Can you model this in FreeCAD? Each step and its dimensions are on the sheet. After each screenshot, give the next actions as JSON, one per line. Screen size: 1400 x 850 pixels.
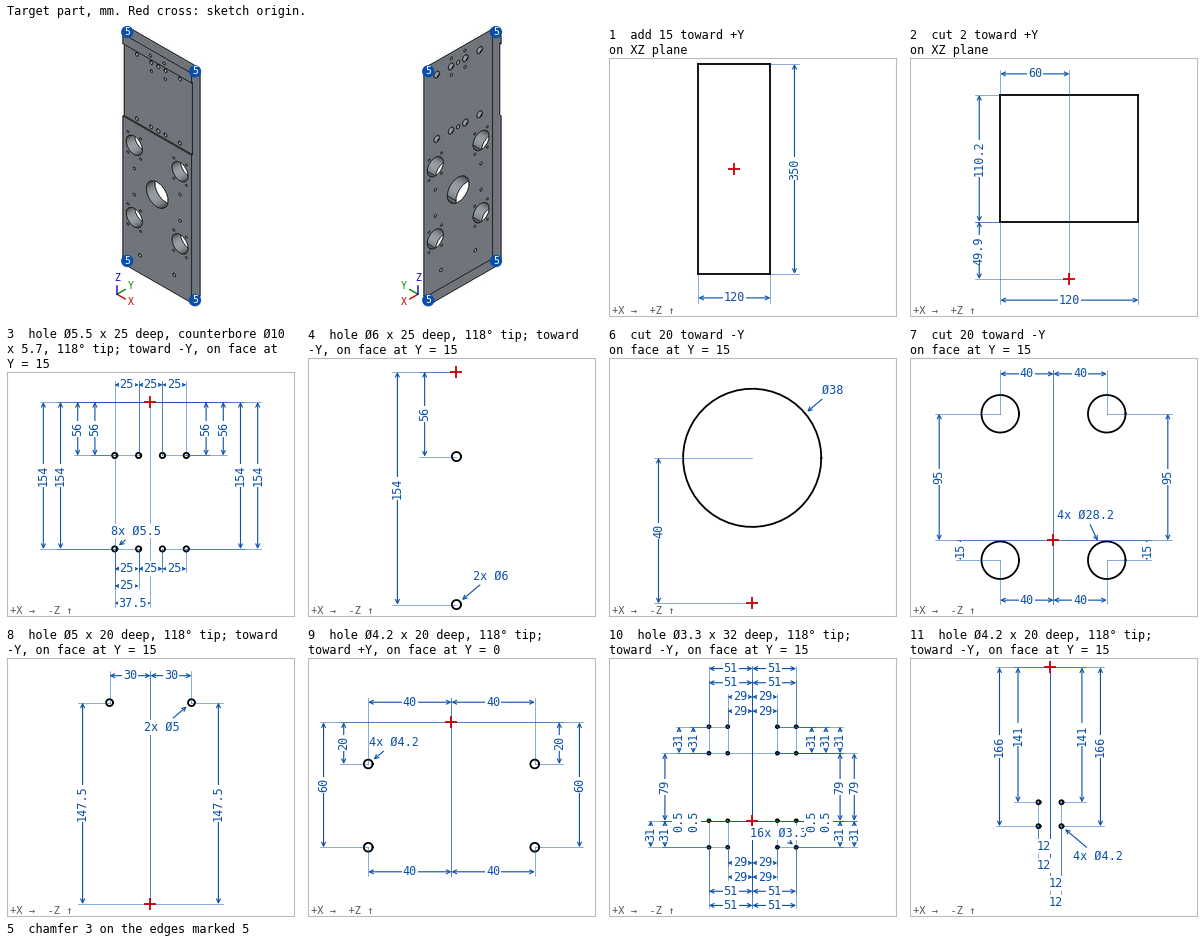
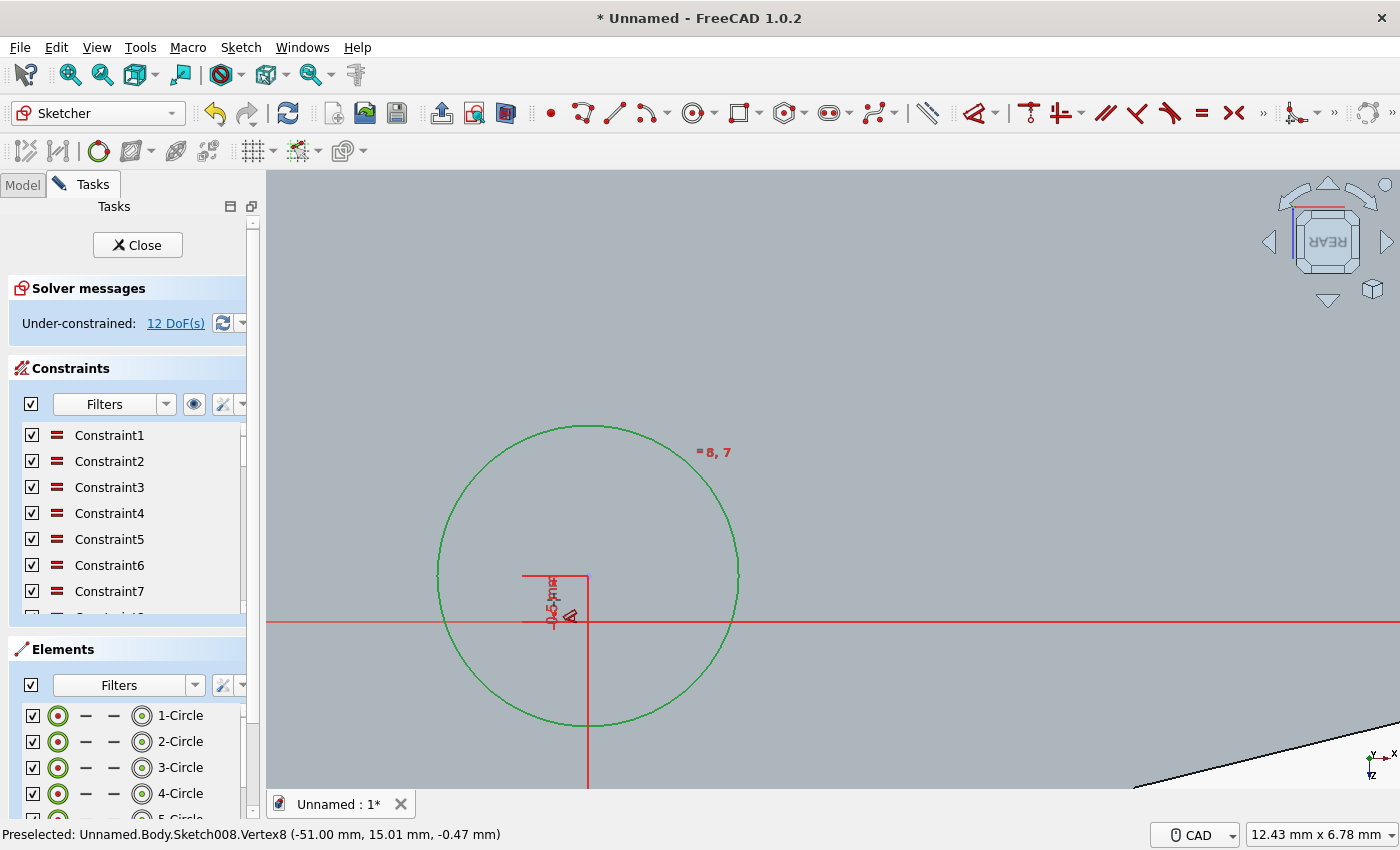
{"action": "scroll", "coordinate": [610, 601], "scroll_direction": "down", "scroll_amount": 17}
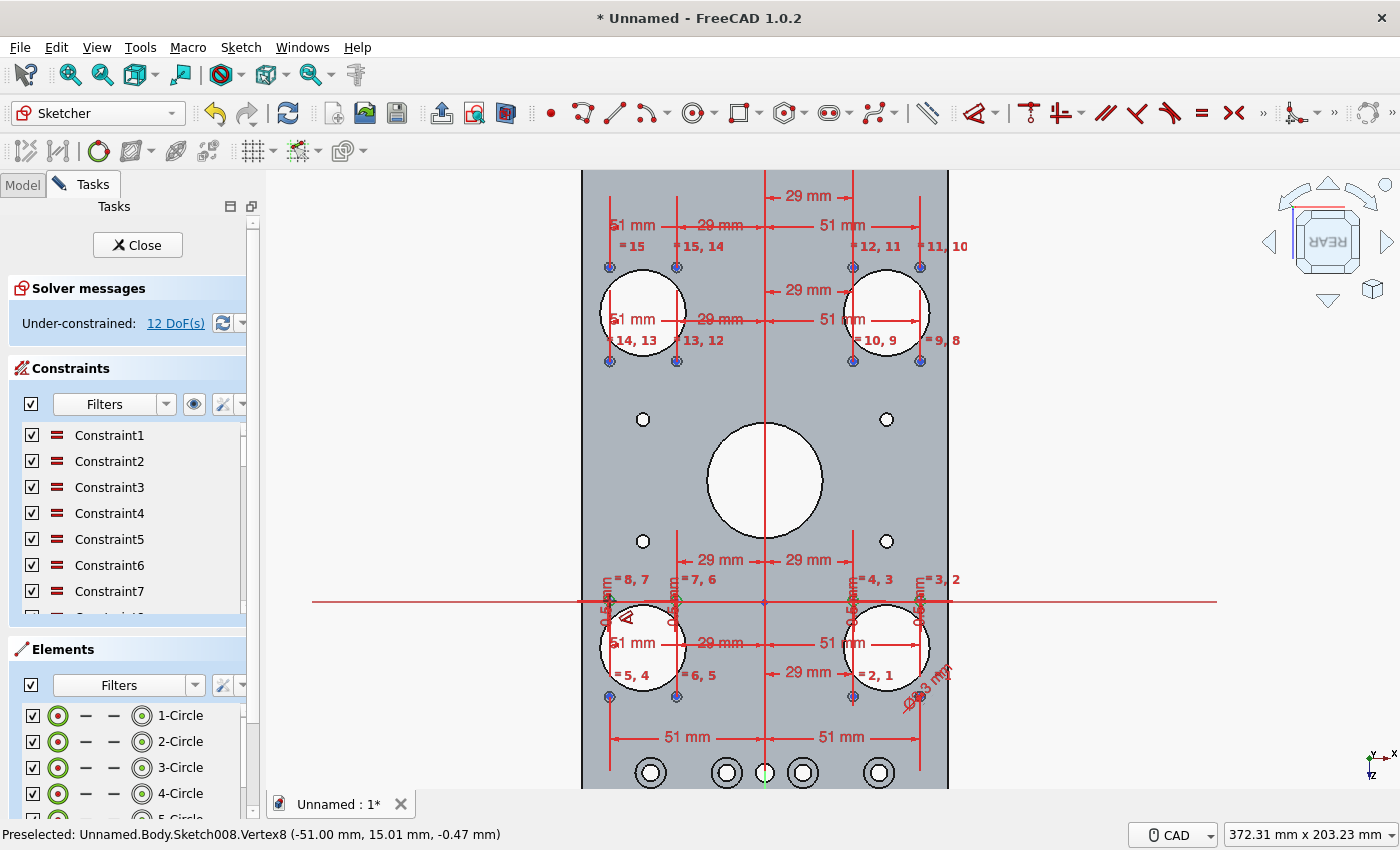
{"action": "left_click", "coordinate": [920, 697]}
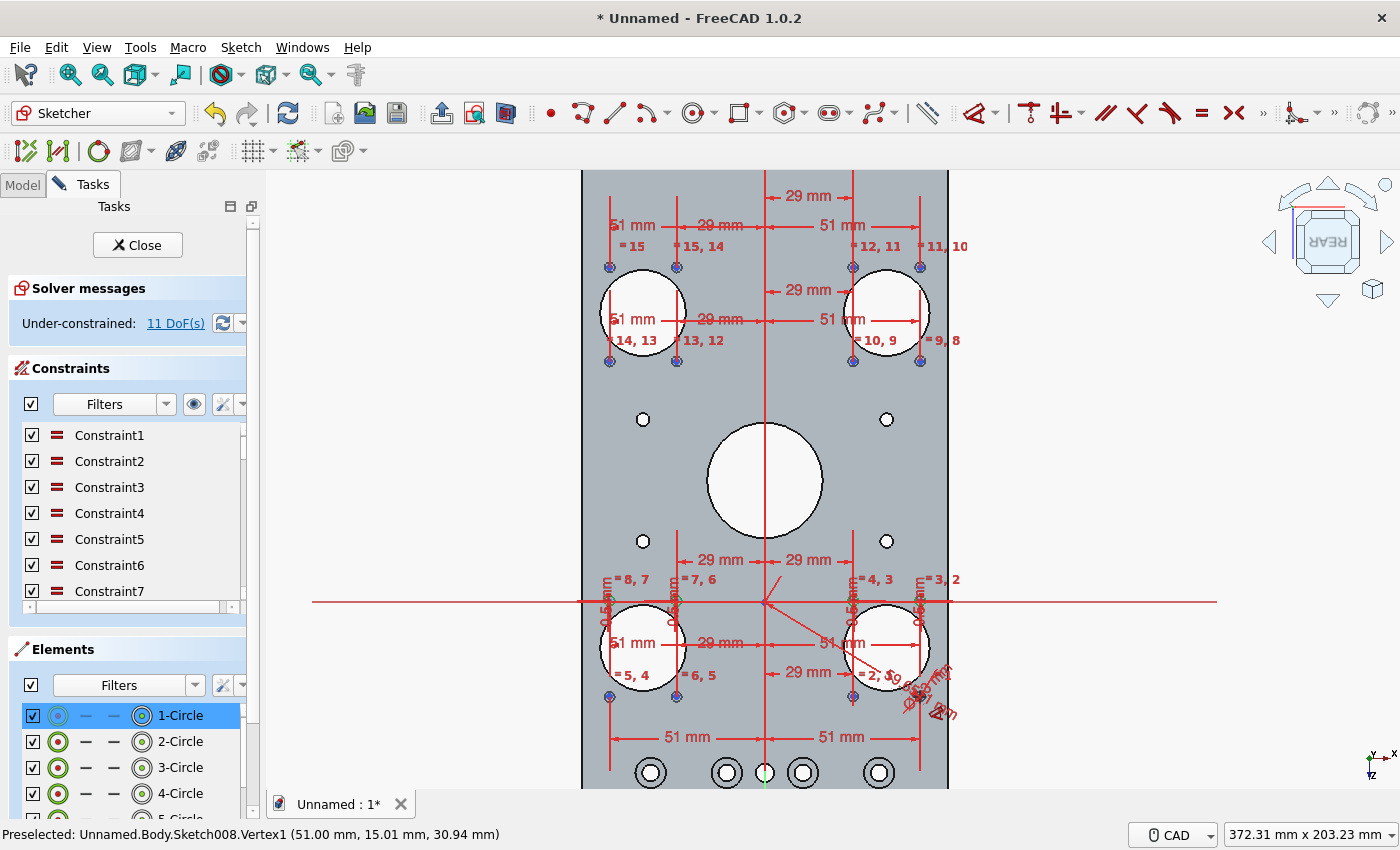
{"action": "left_click", "coordinate": [920, 601]}
{"action": "left_click", "coordinate": [954, 649]}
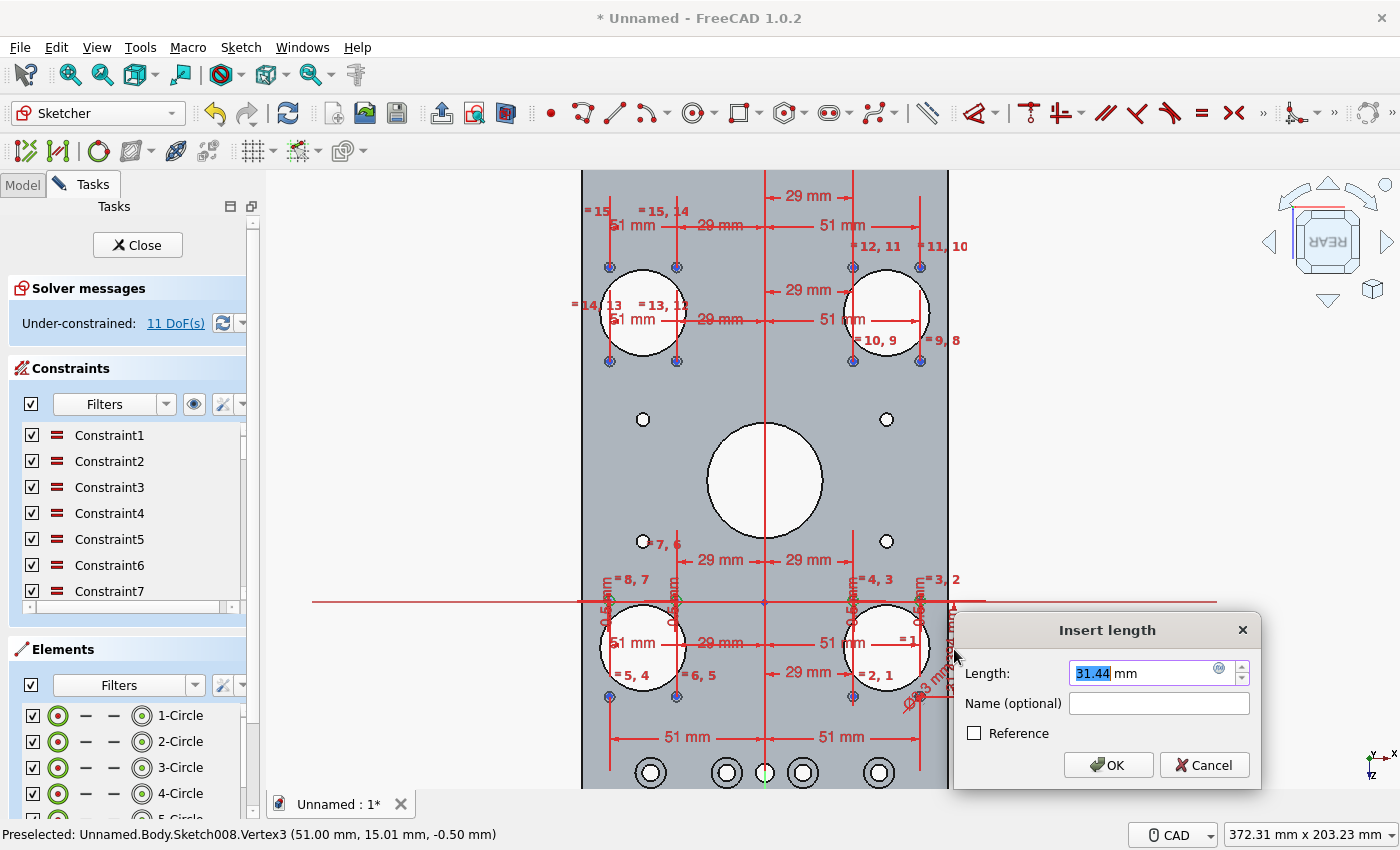
{"action": "type", "text": "31"}
{"action": "key", "text": "Return"}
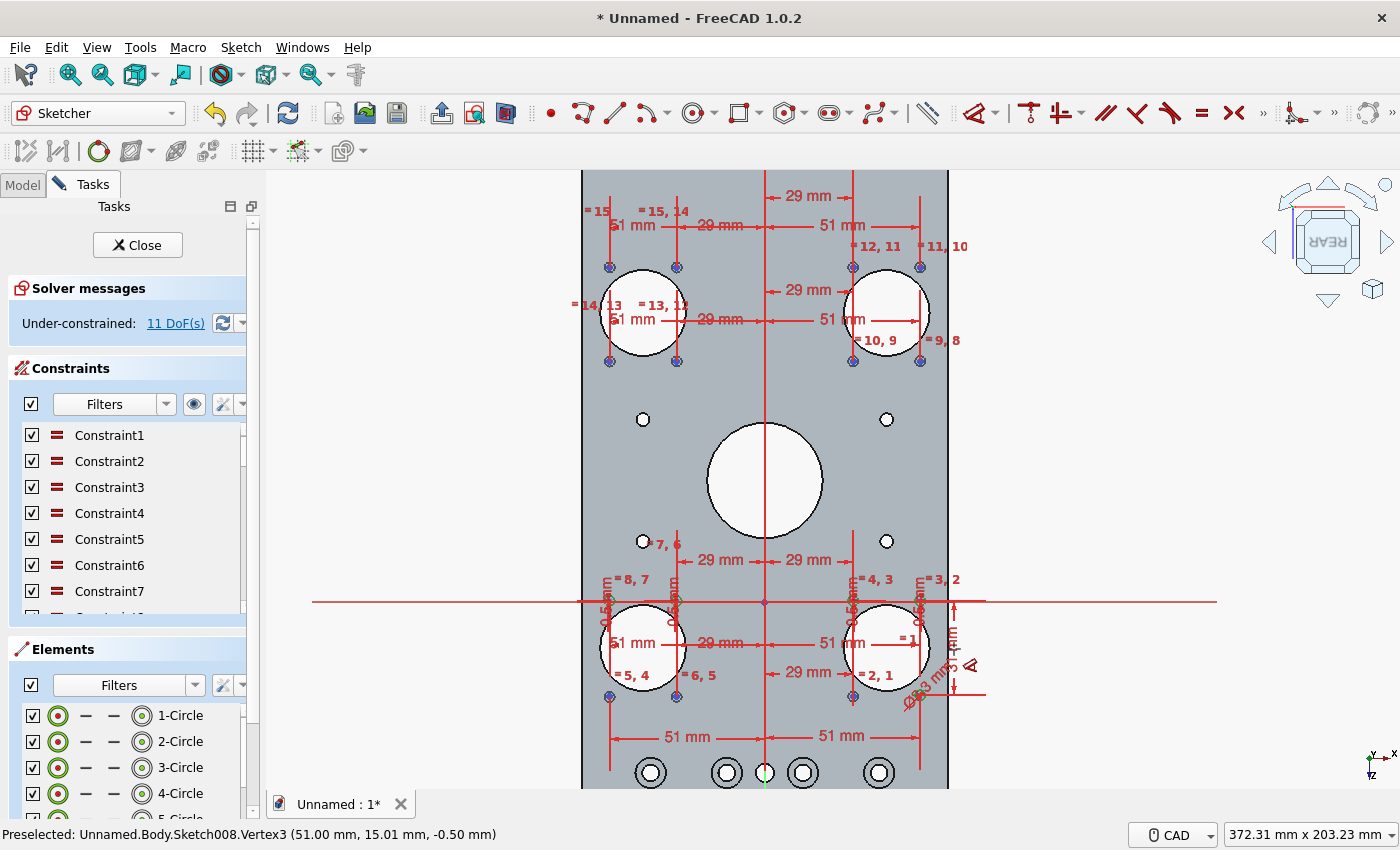
{"action": "left_click", "coordinate": [853, 696]}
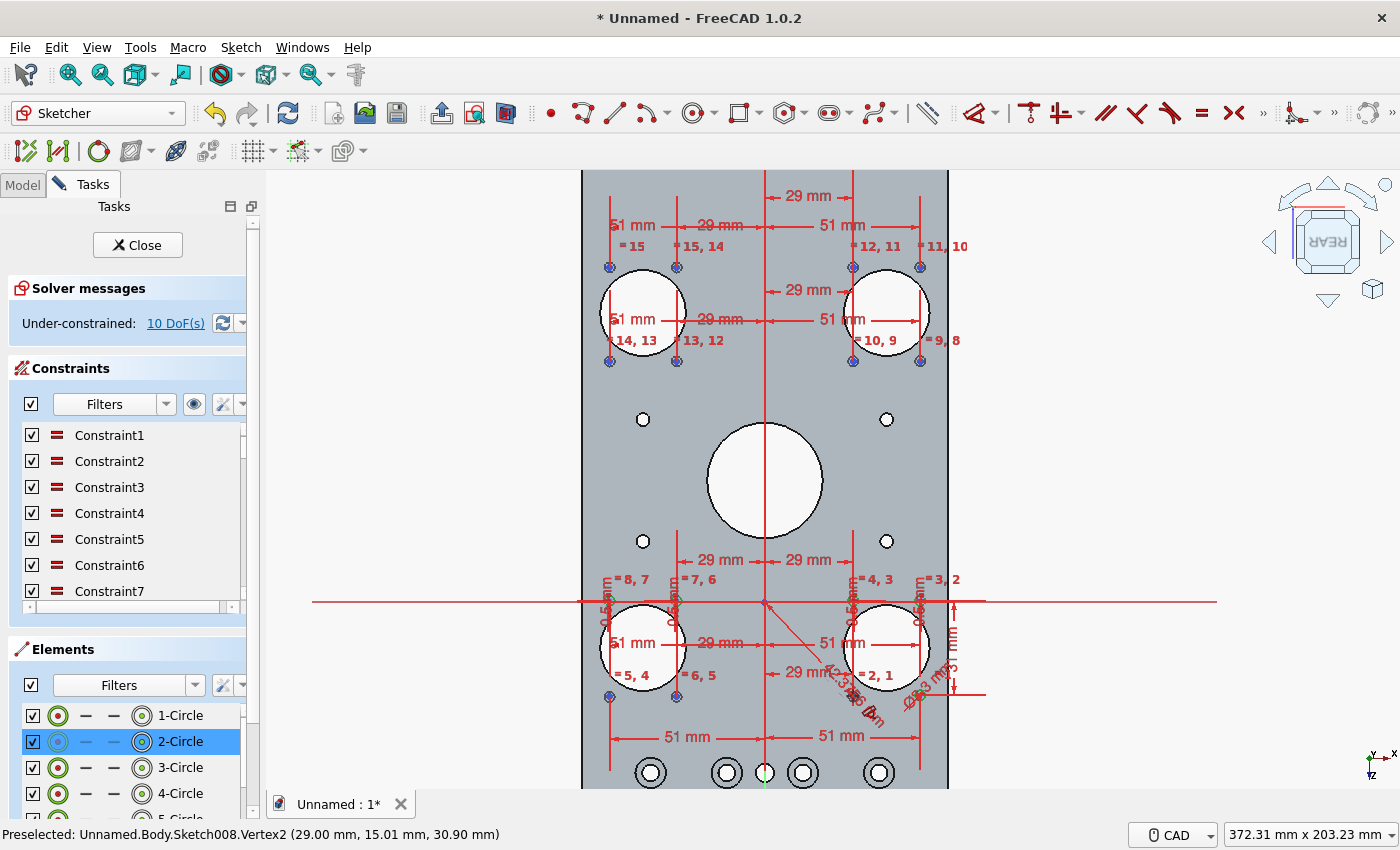
{"action": "left_click", "coordinate": [920, 601]}
{"action": "left_click", "coordinate": [954, 627]}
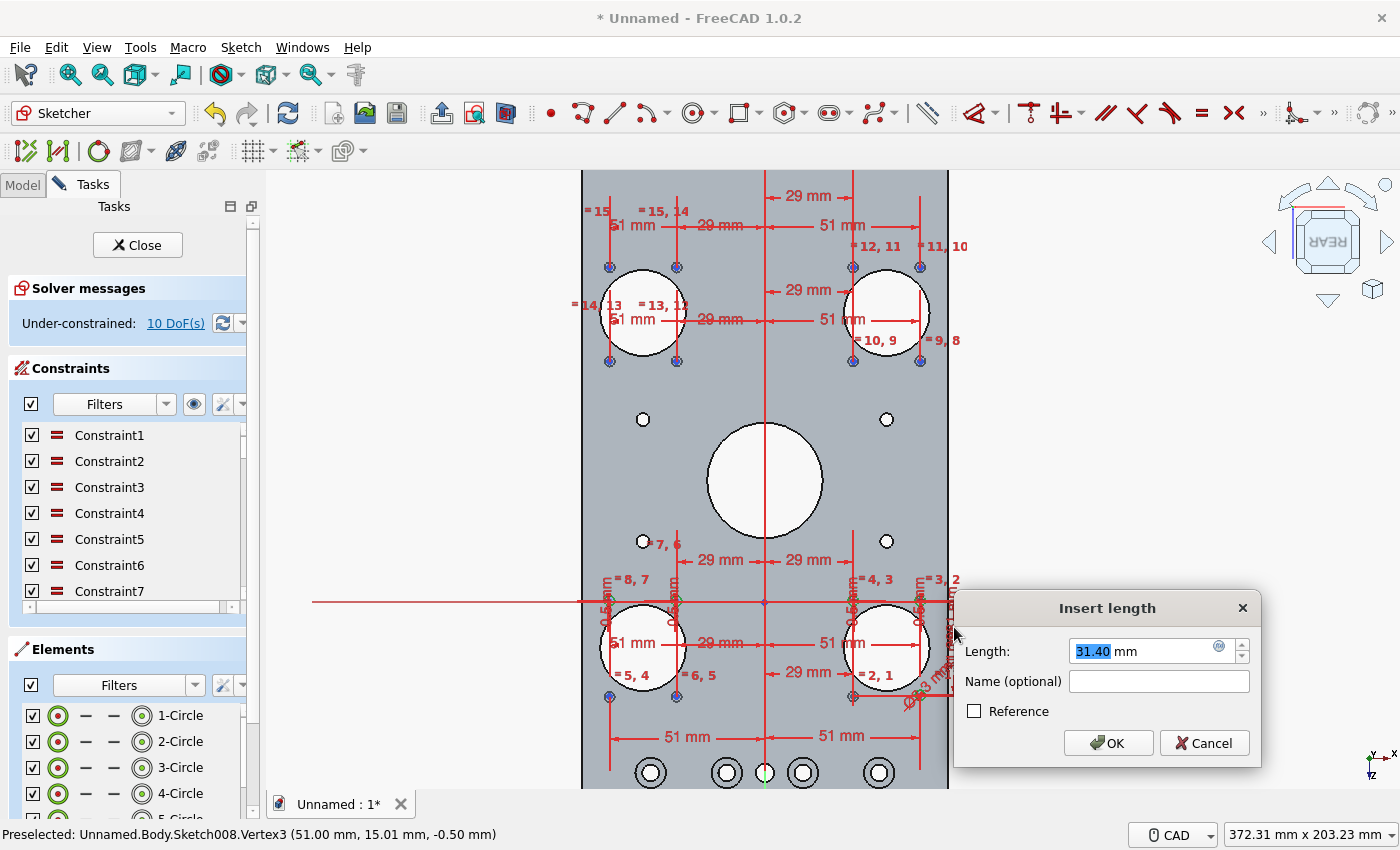
{"action": "type", "text": "31"}
{"action": "key", "text": "Return"}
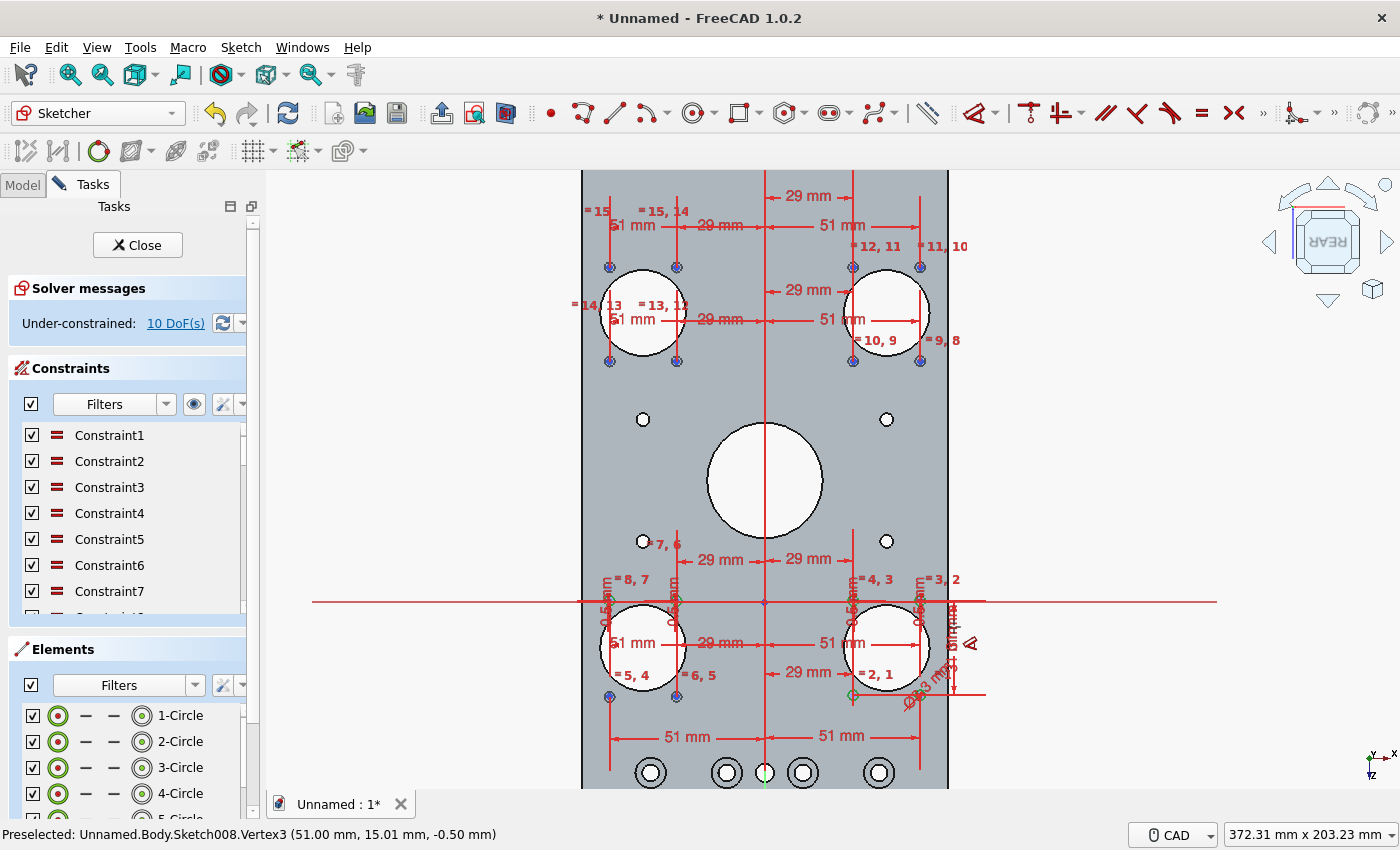
{"action": "left_click", "coordinate": [853, 601]}